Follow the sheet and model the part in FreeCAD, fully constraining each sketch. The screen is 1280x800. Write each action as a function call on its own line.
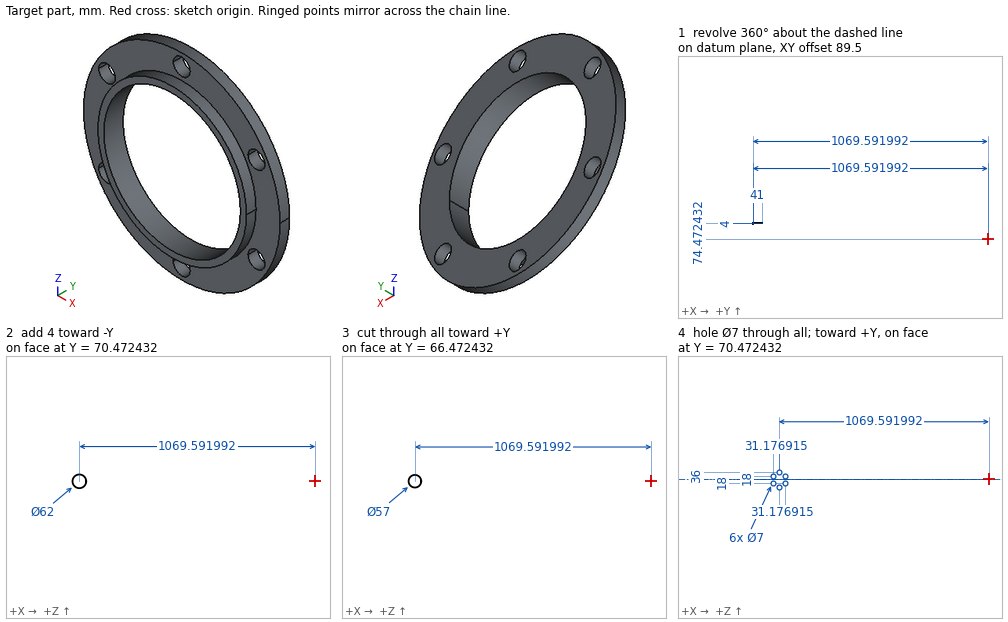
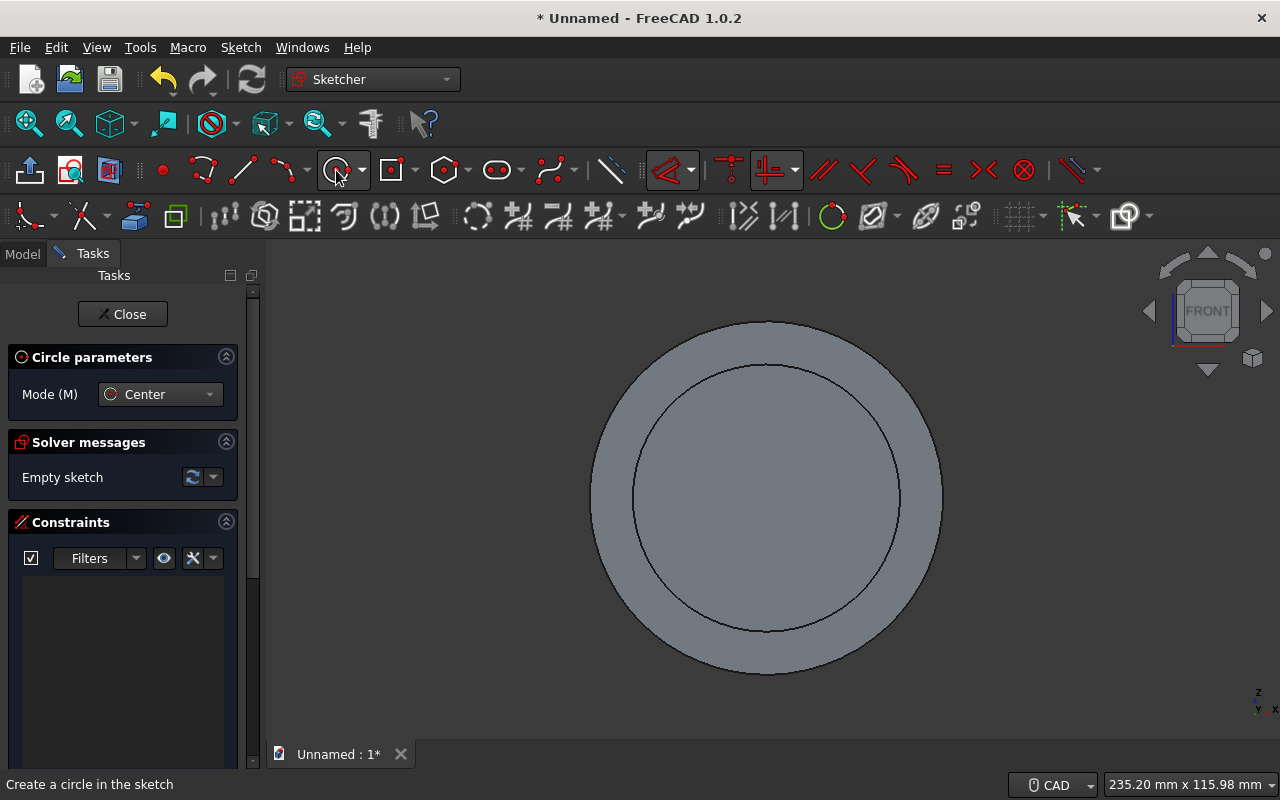
click(766, 498)
move(853, 411)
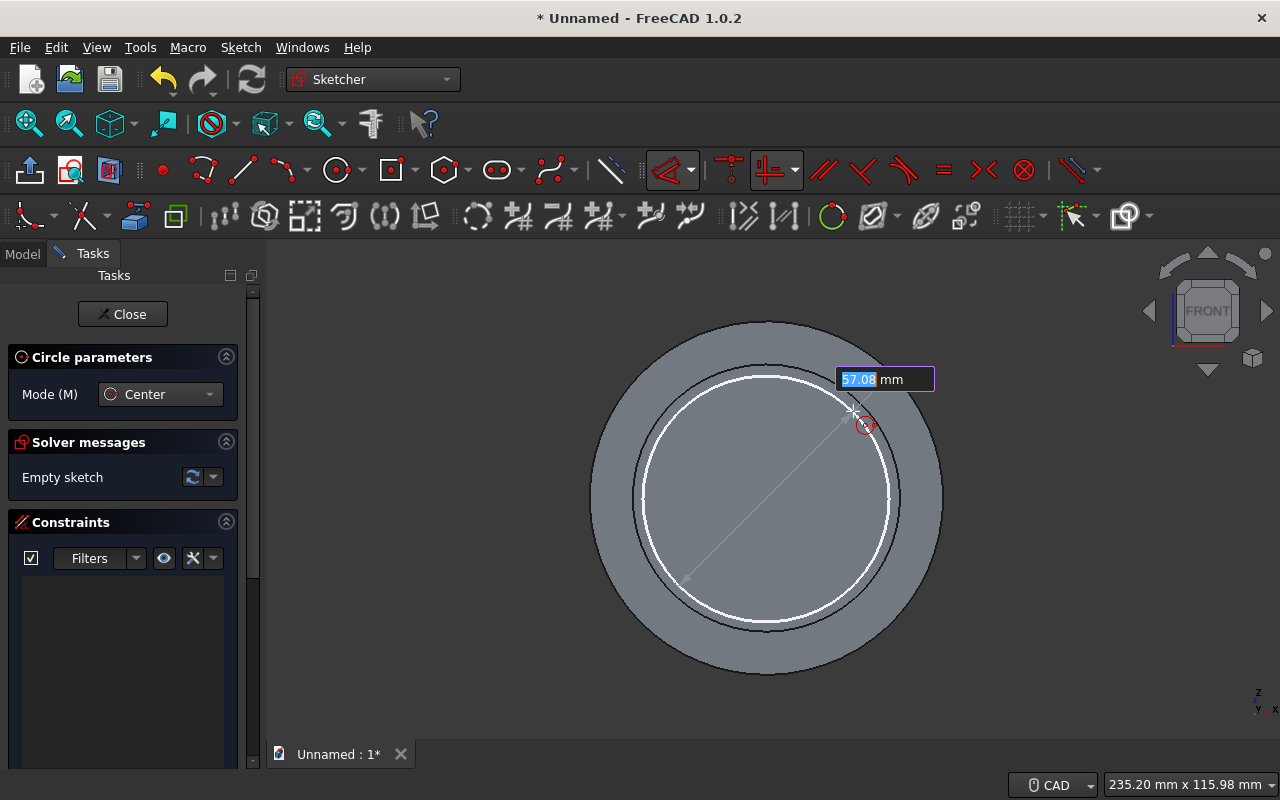
text(57)
key(Return)
key(Escape)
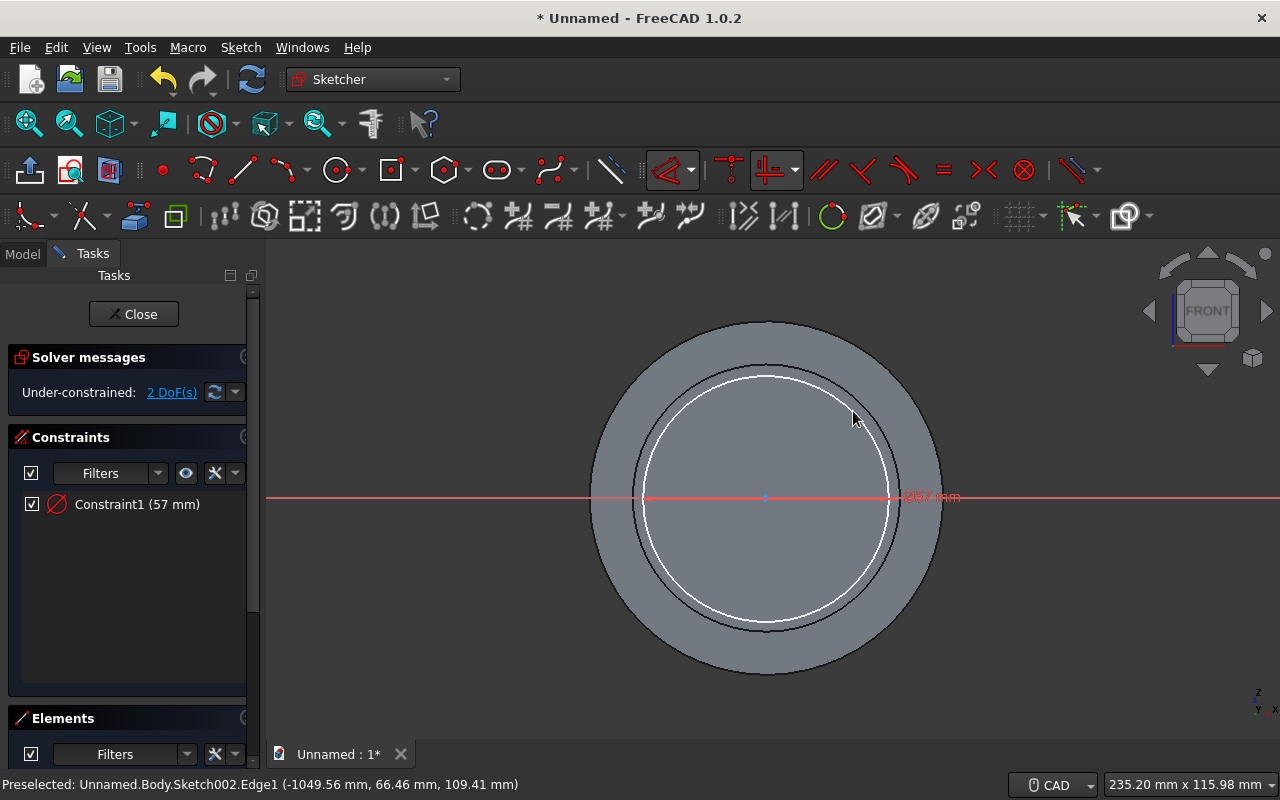
click(766, 499)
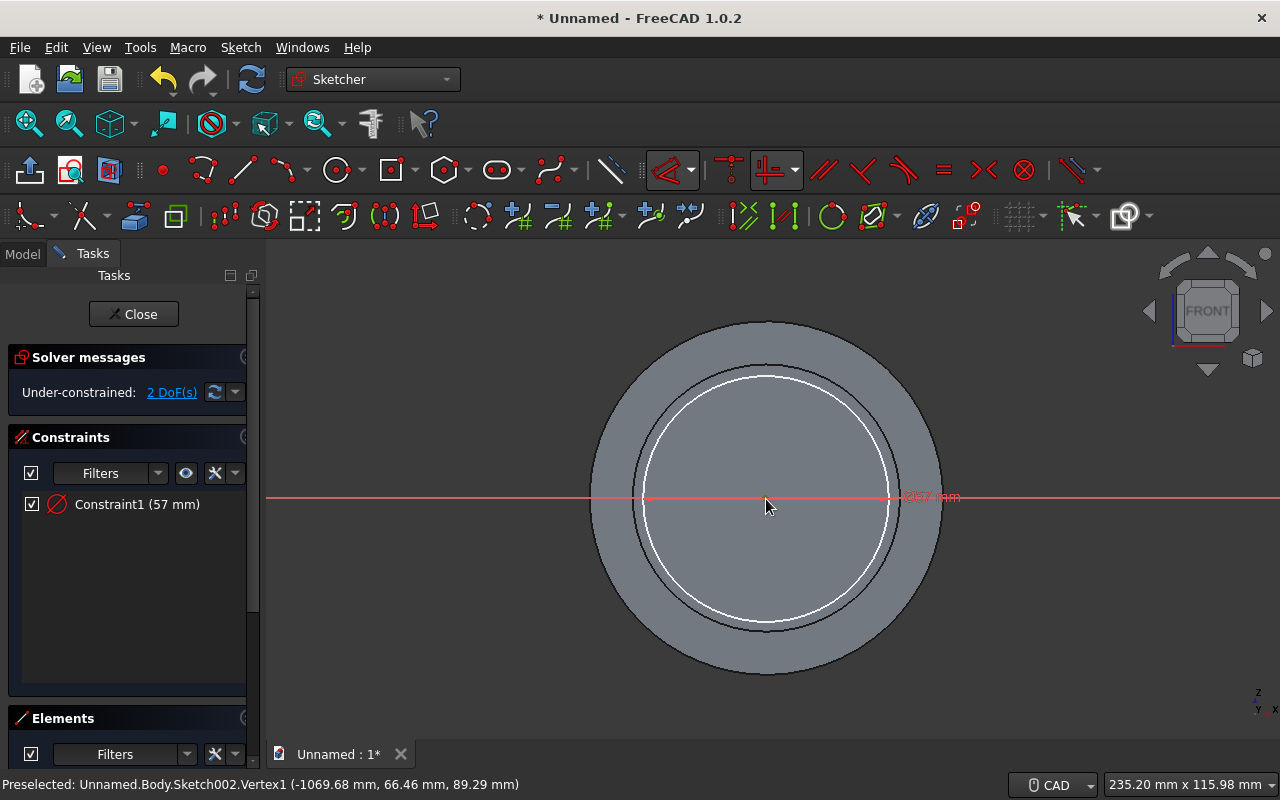
click(353, 498)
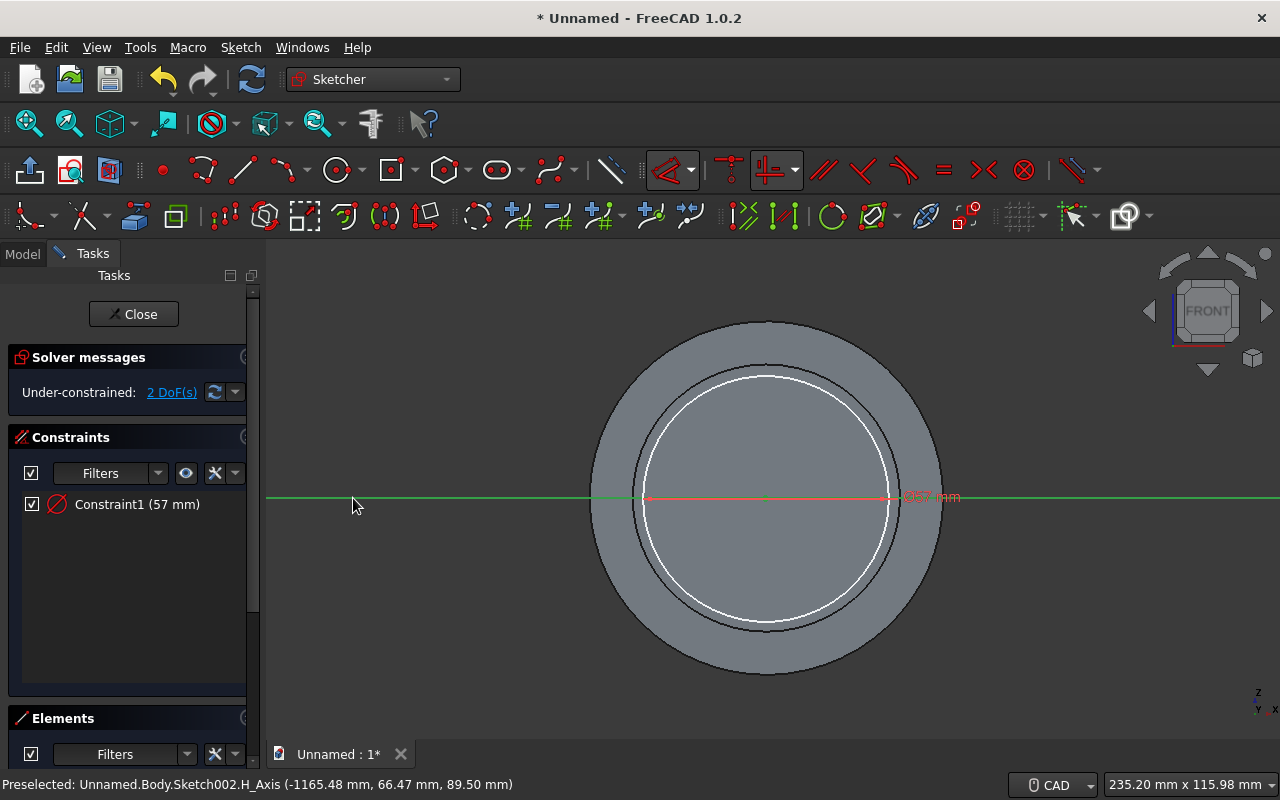
click(730, 170)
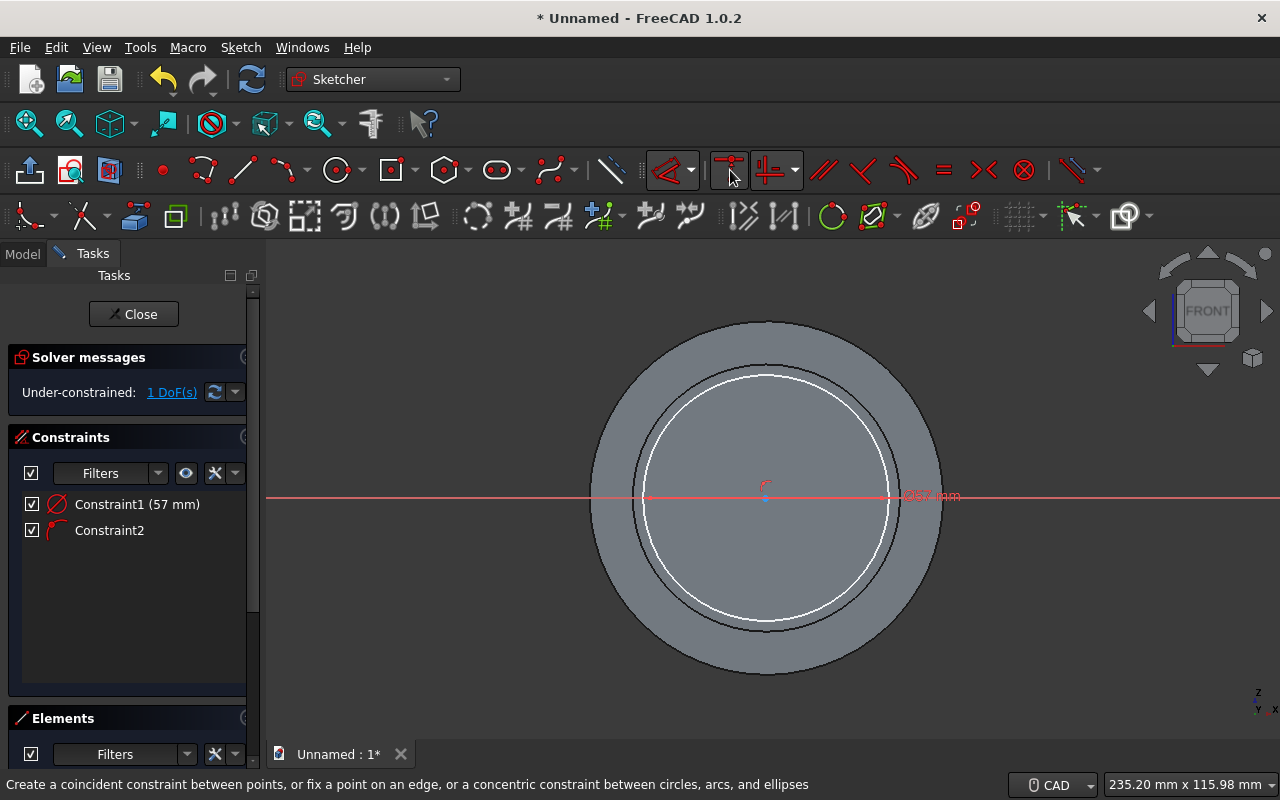
click(766, 498)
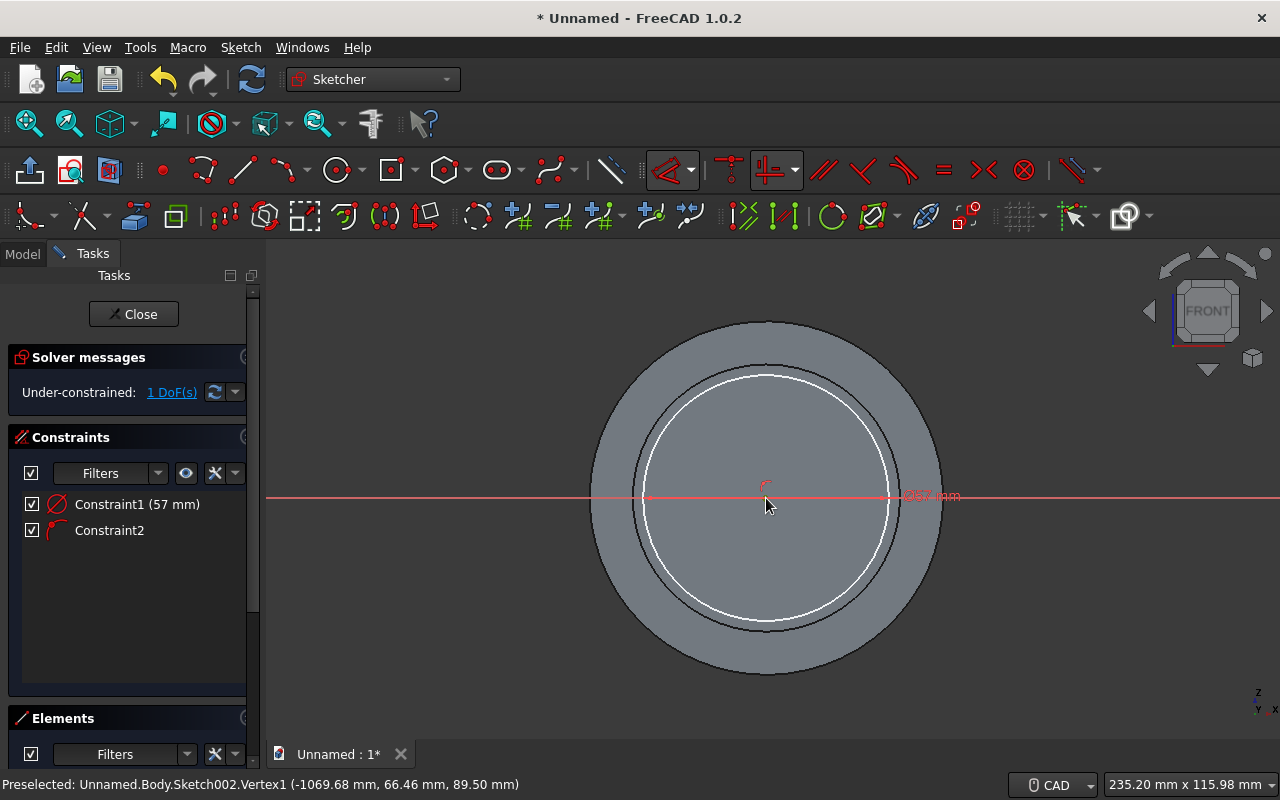
key(l)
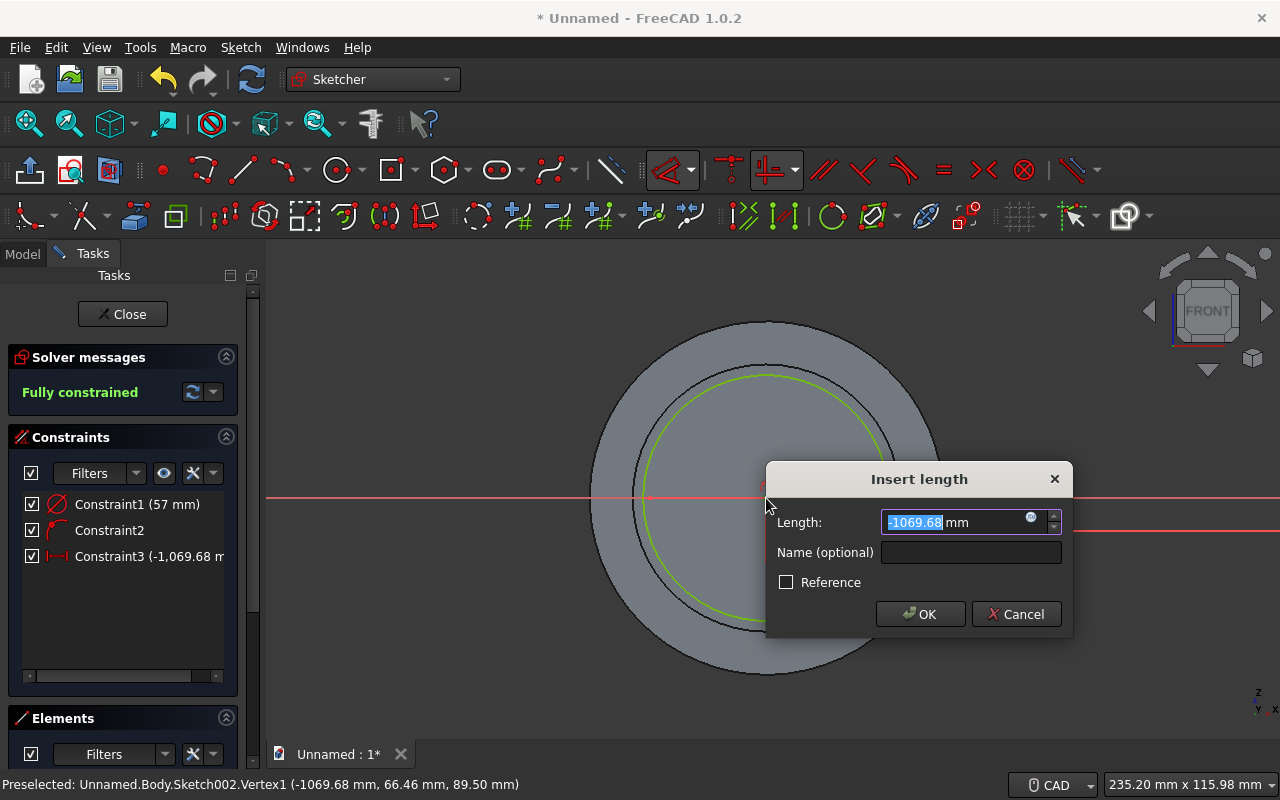
text(-1069.591992)
key(Return)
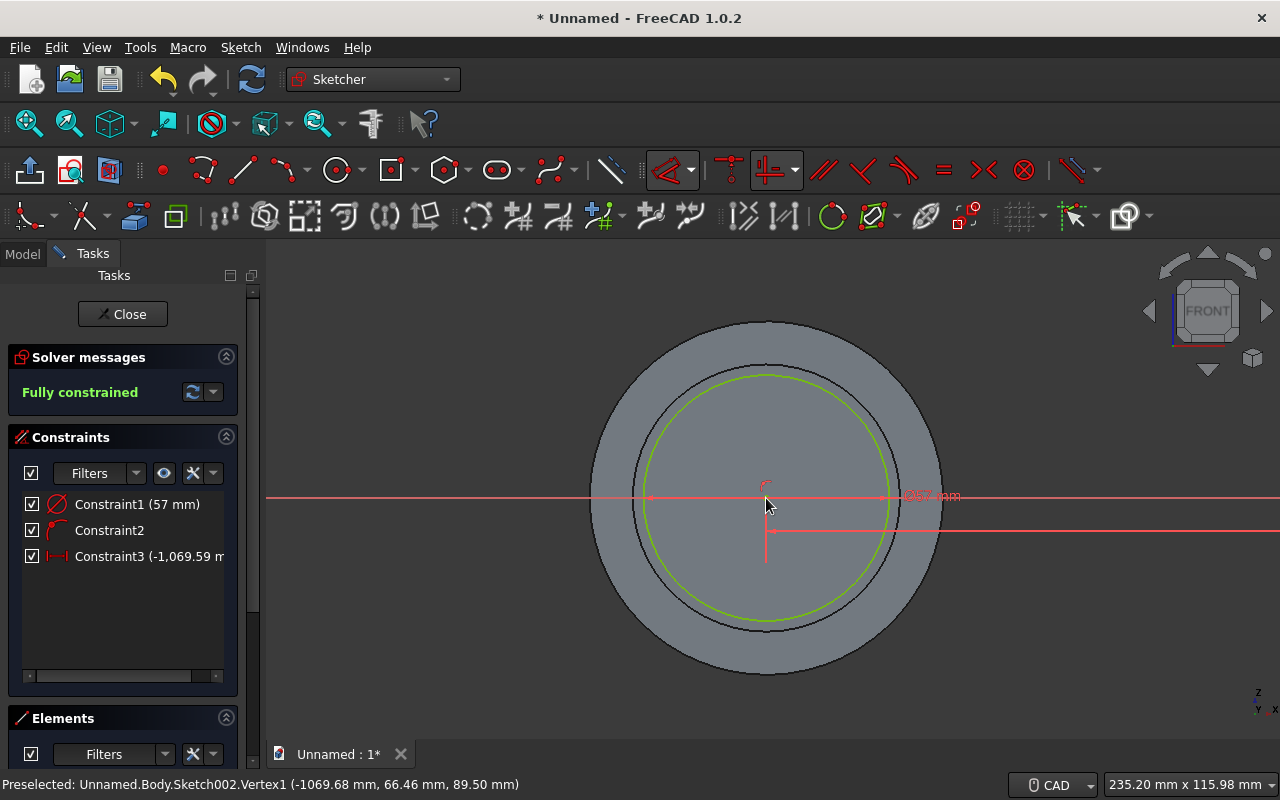
click(123, 314)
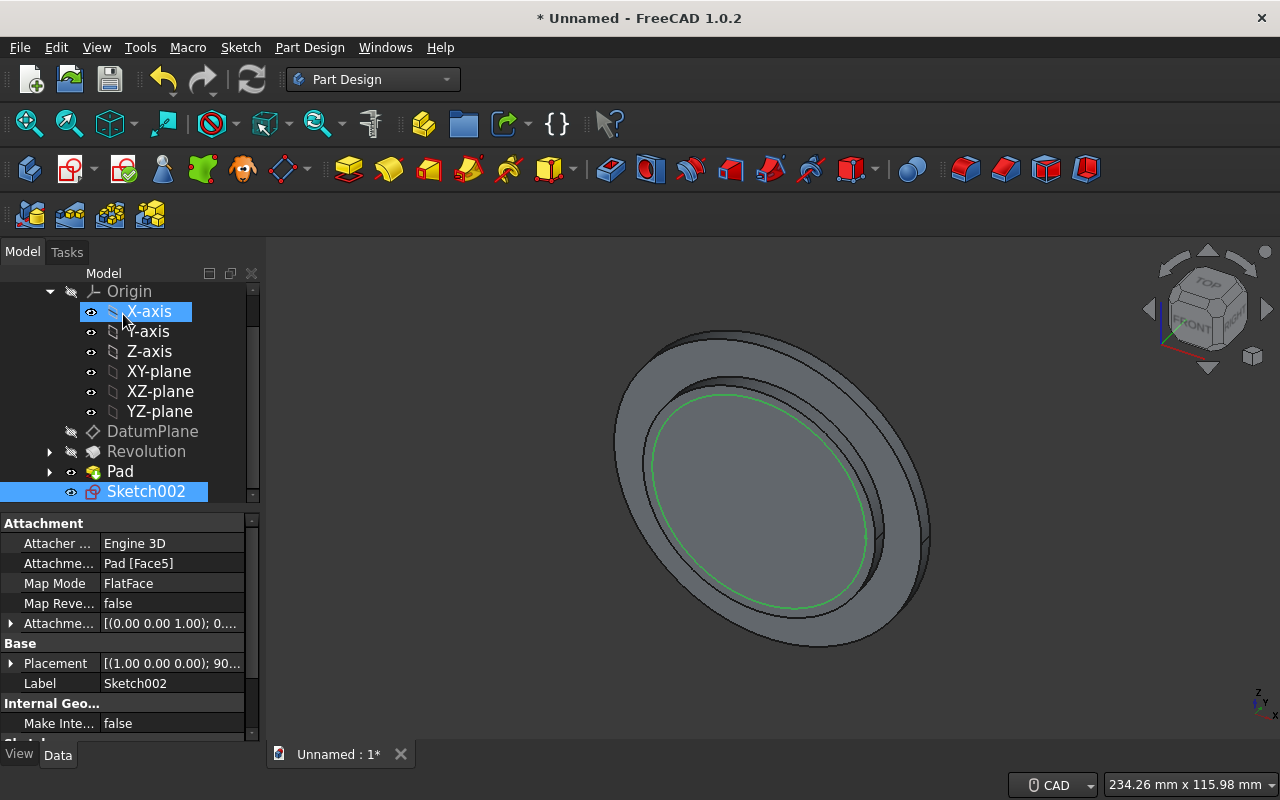
click(612, 170)